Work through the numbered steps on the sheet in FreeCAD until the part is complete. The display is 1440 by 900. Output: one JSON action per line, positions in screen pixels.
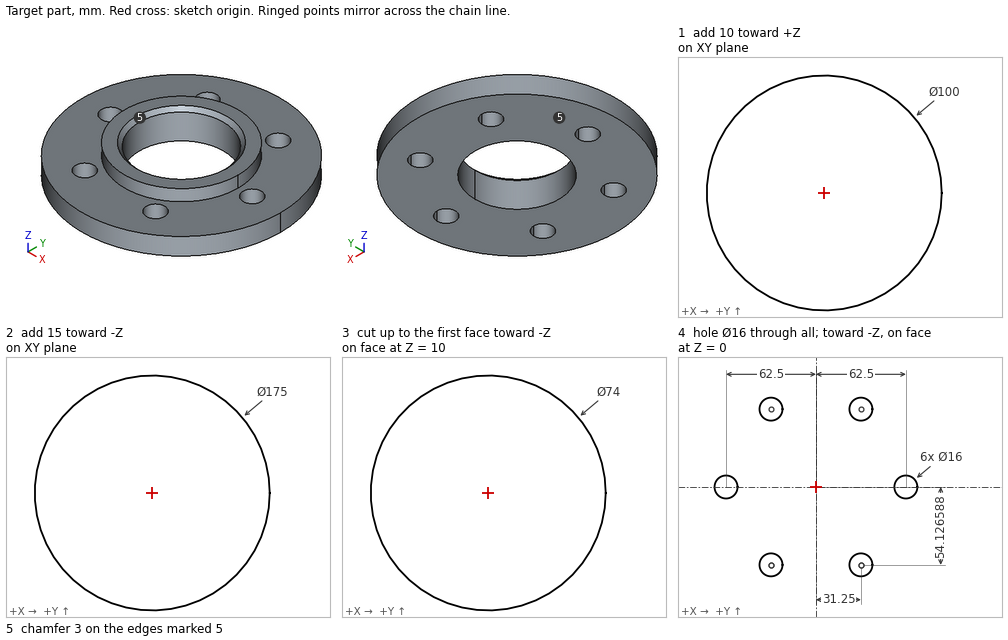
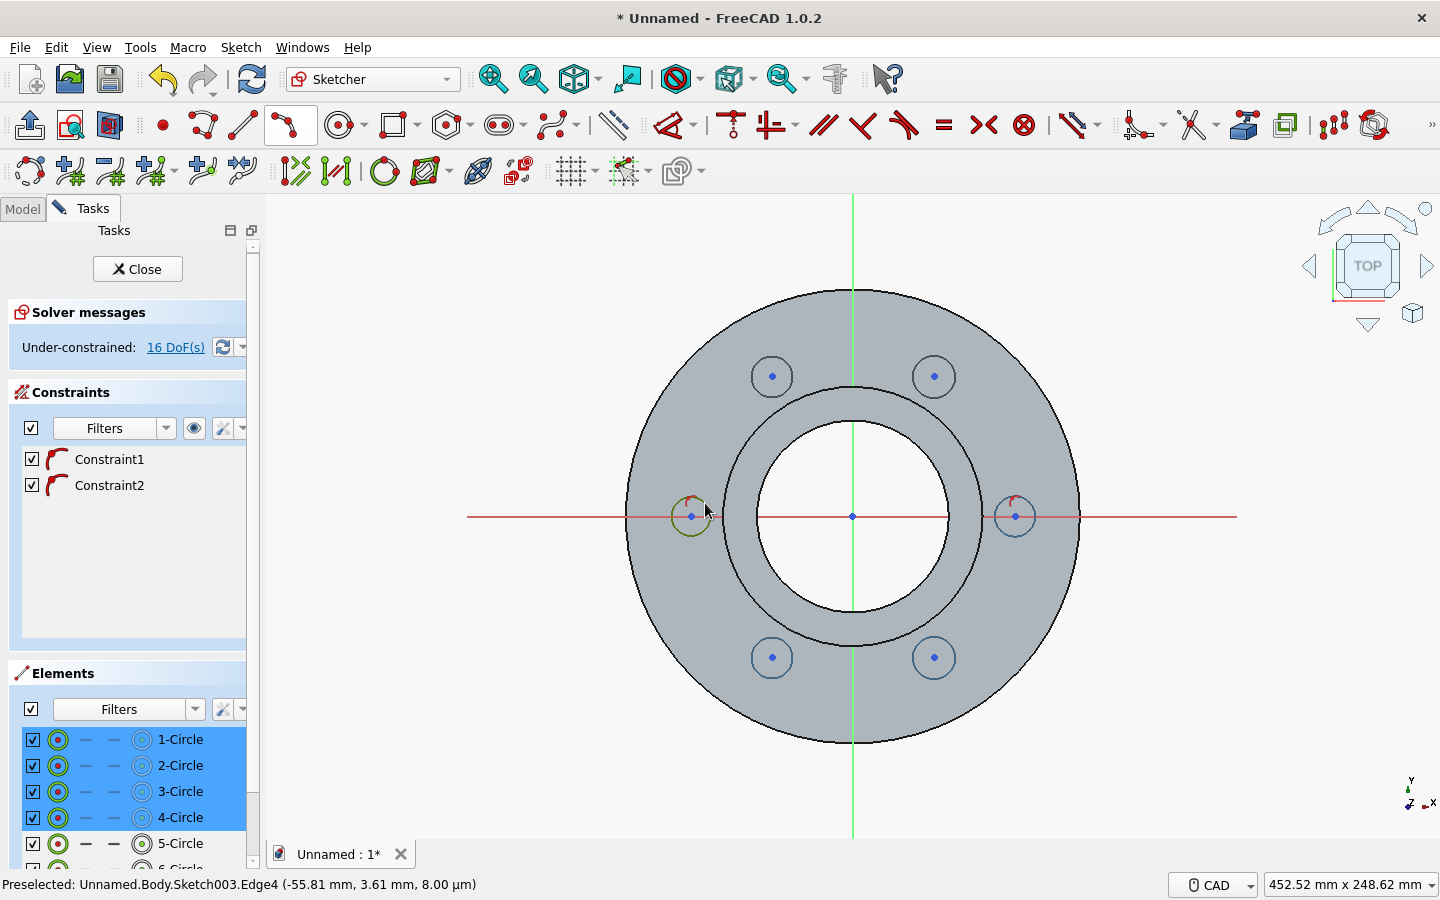
{"action": "left_click", "coordinate": [786, 362]}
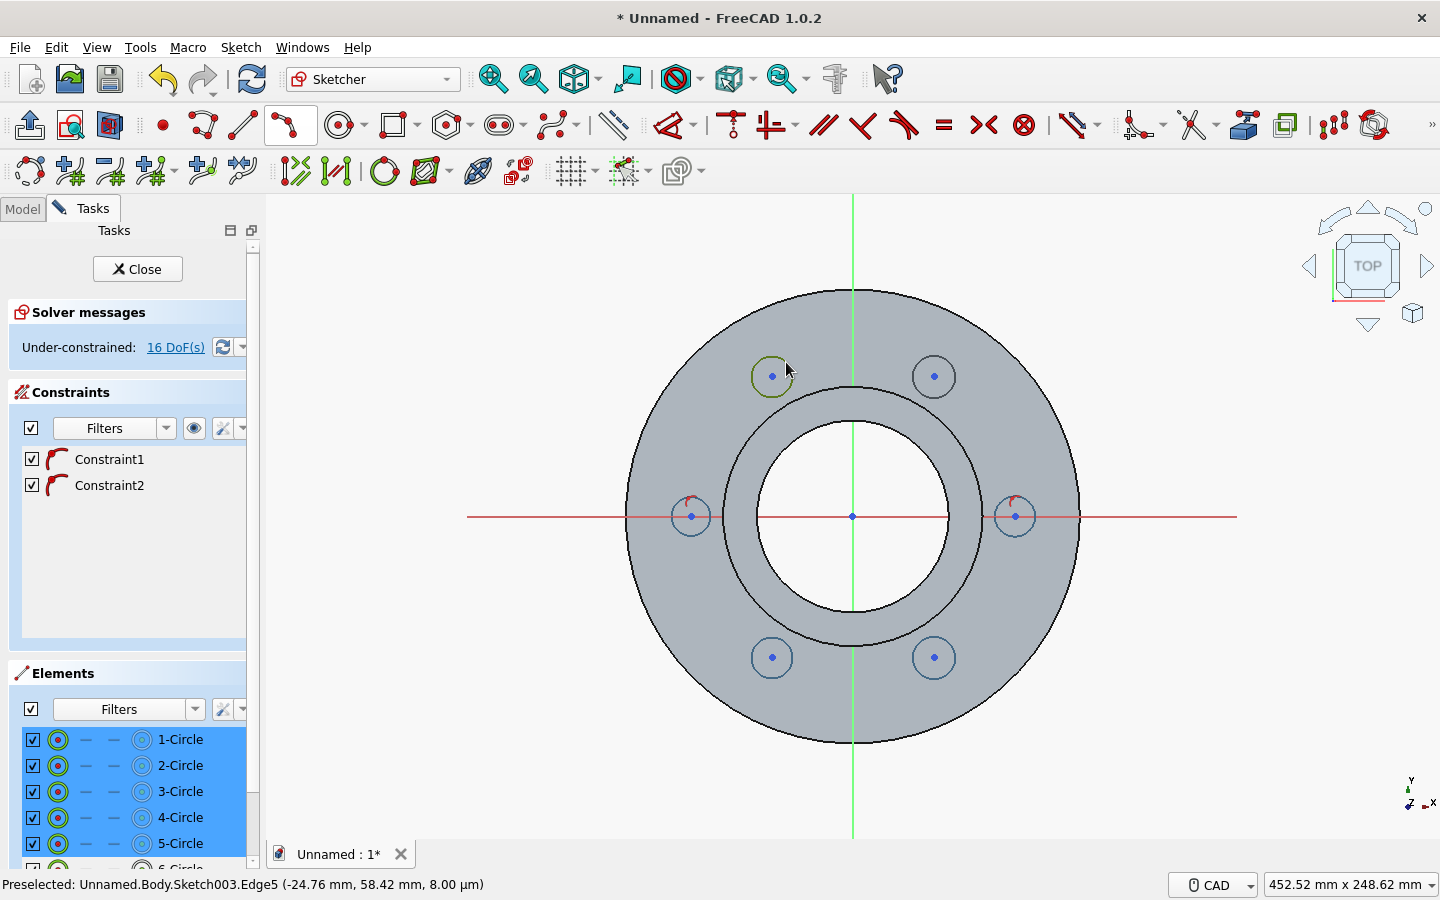
{"action": "left_click", "coordinate": [949, 362]}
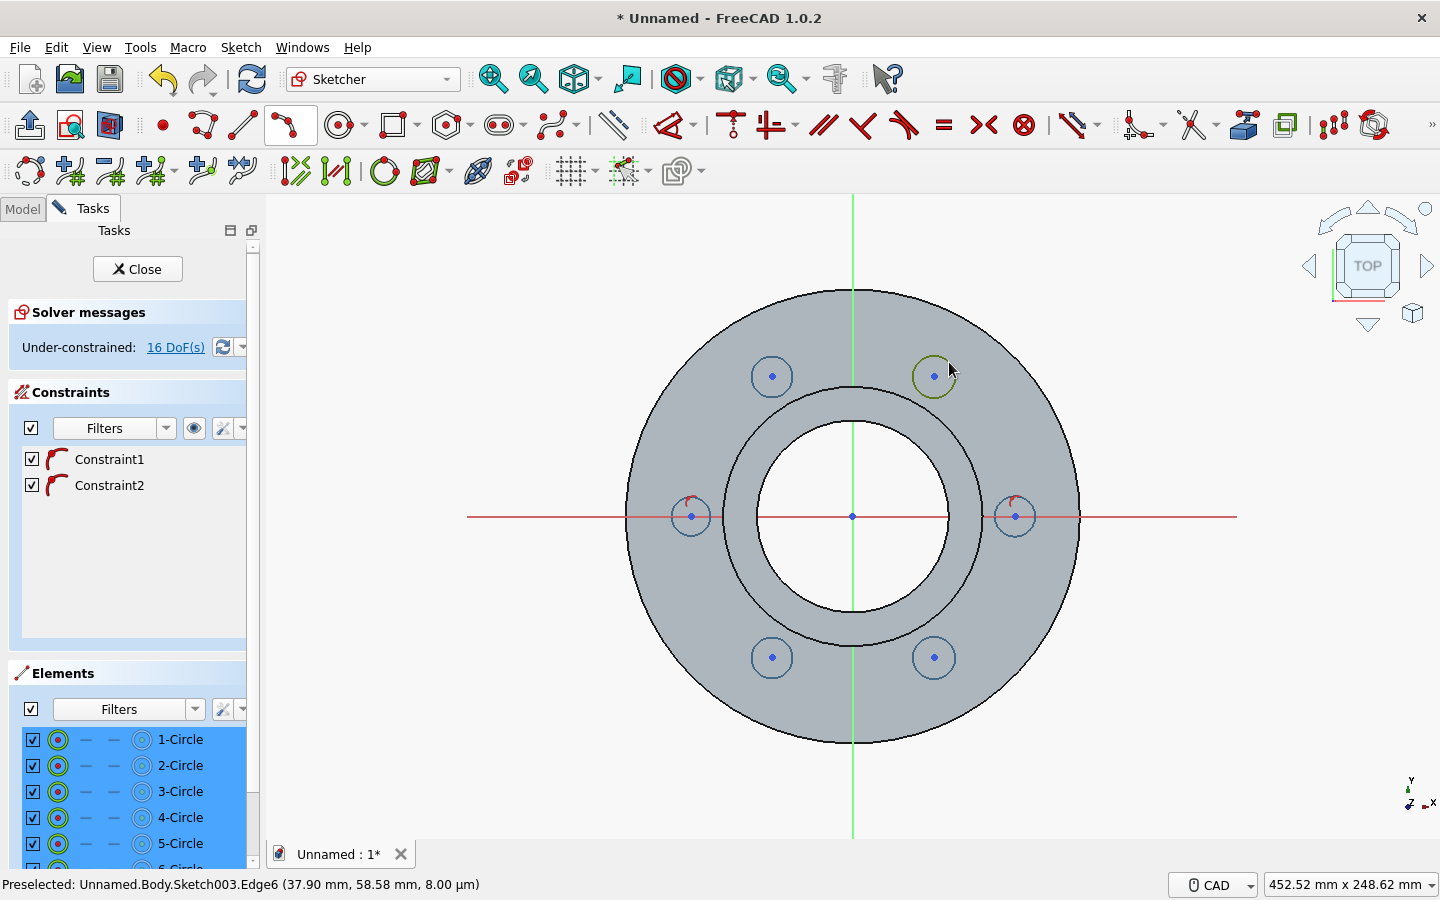
{"action": "key", "text": "e"}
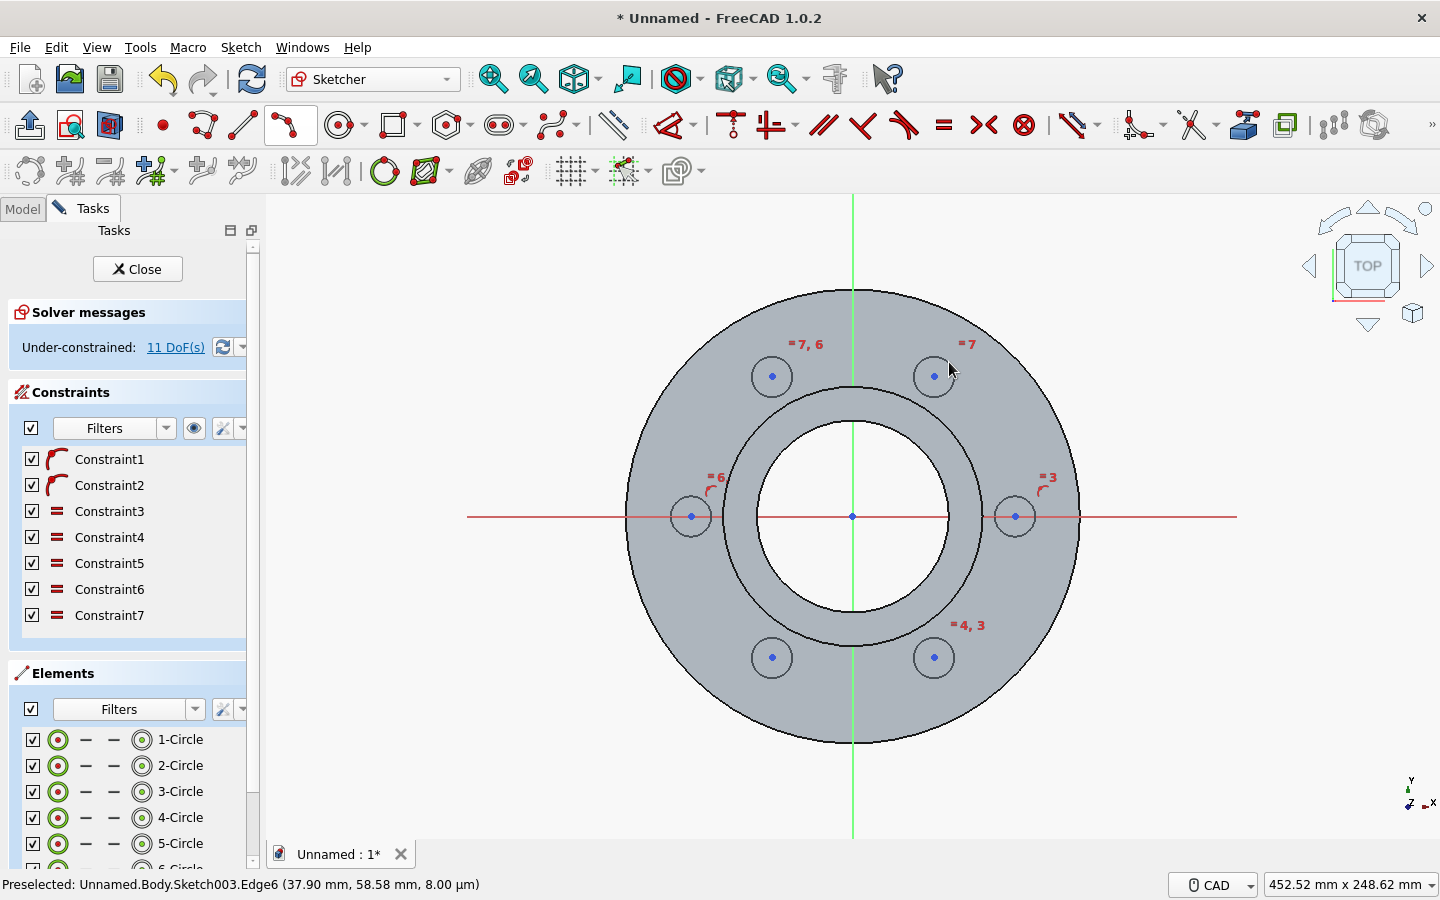
{"action": "left_click", "coordinate": [934, 658]}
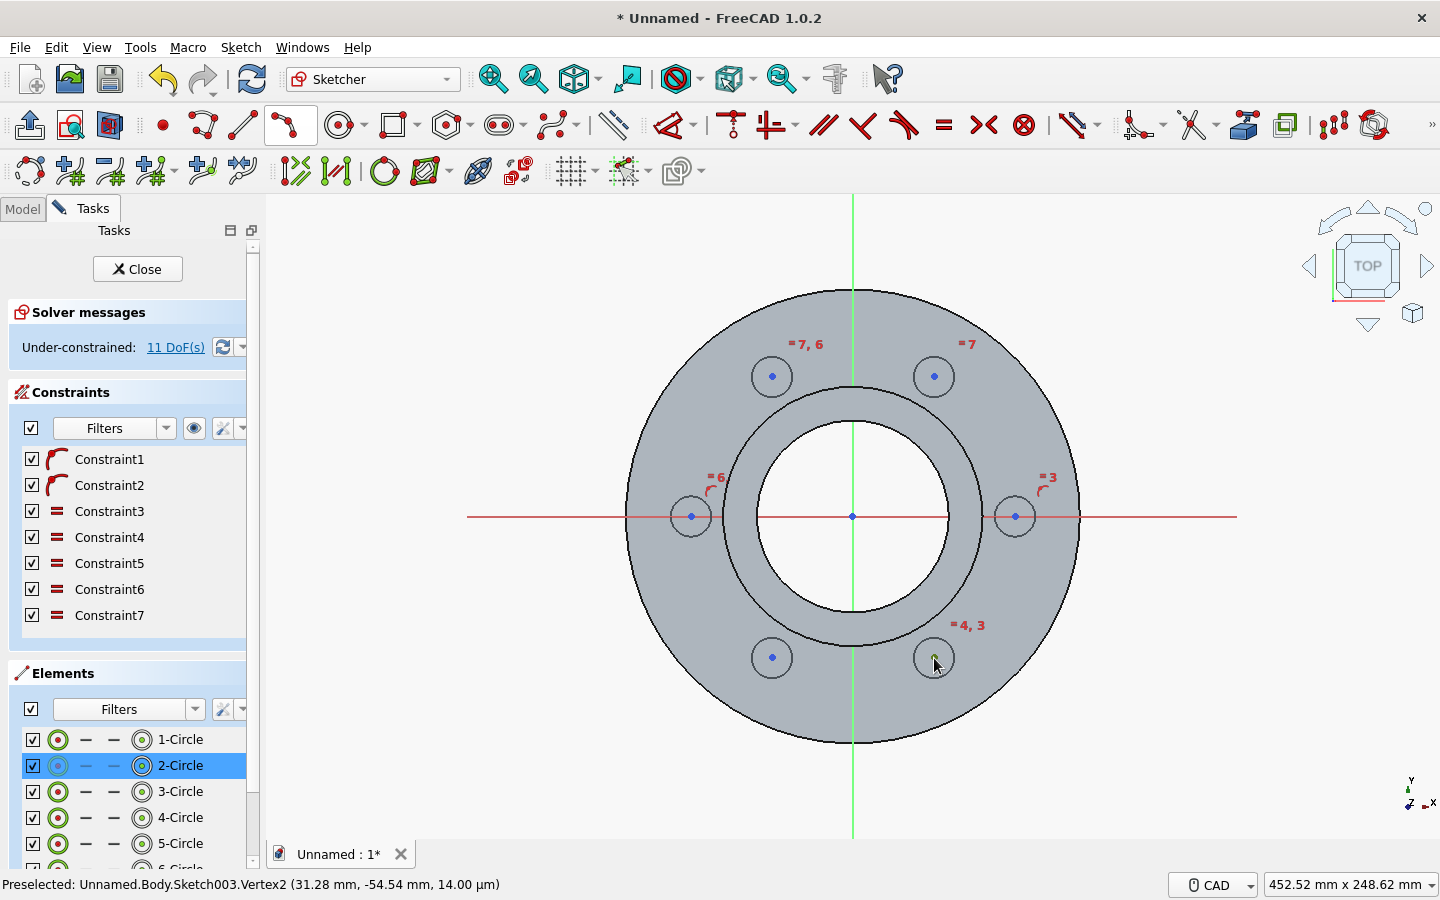
{"action": "left_click", "coordinate": [772, 658]}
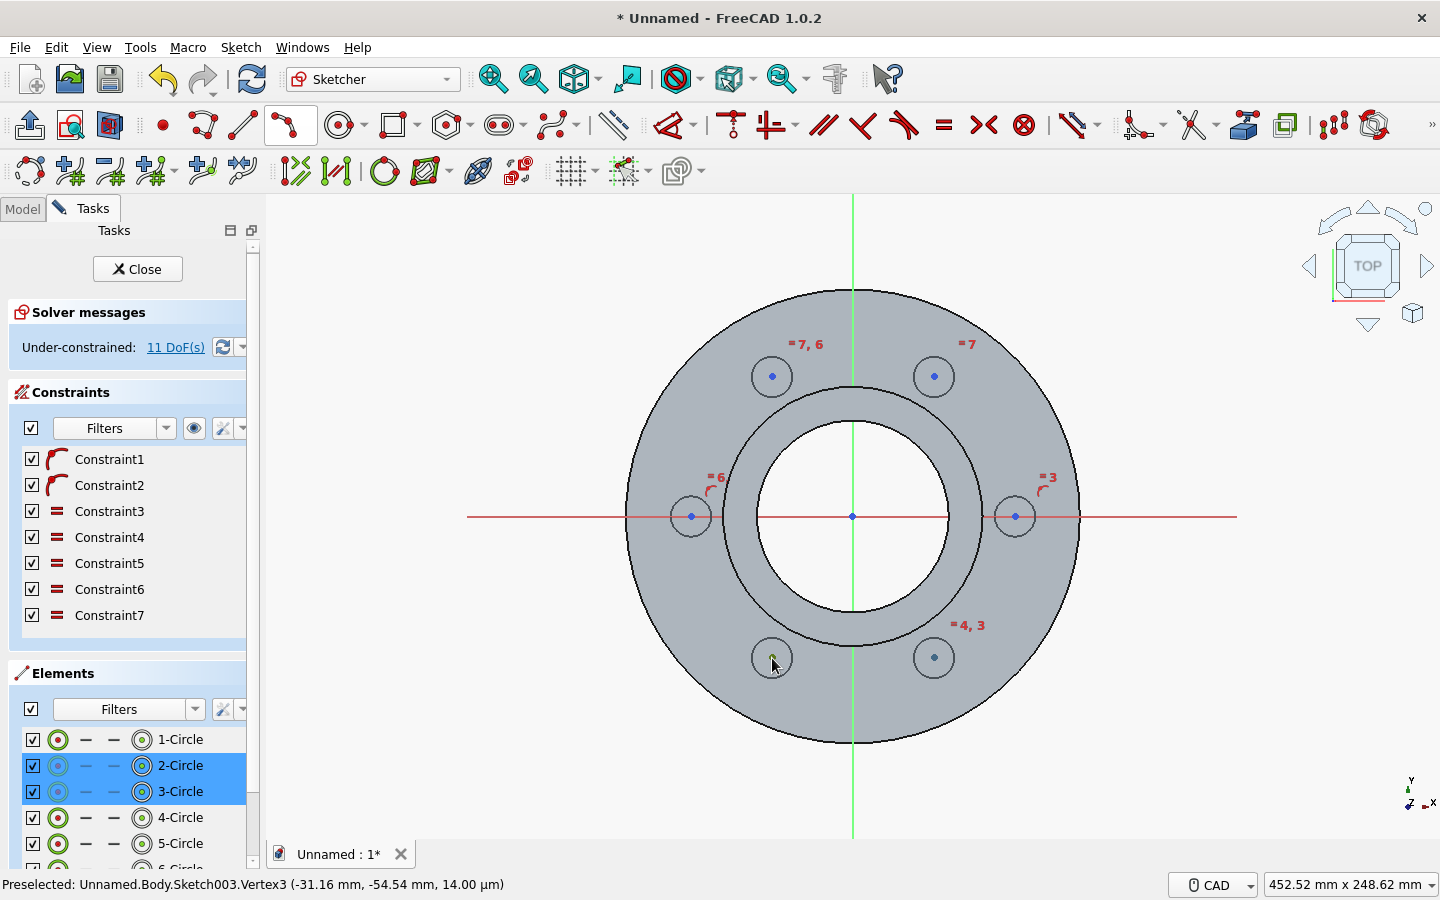
{"action": "left_click", "coordinate": [853, 769]}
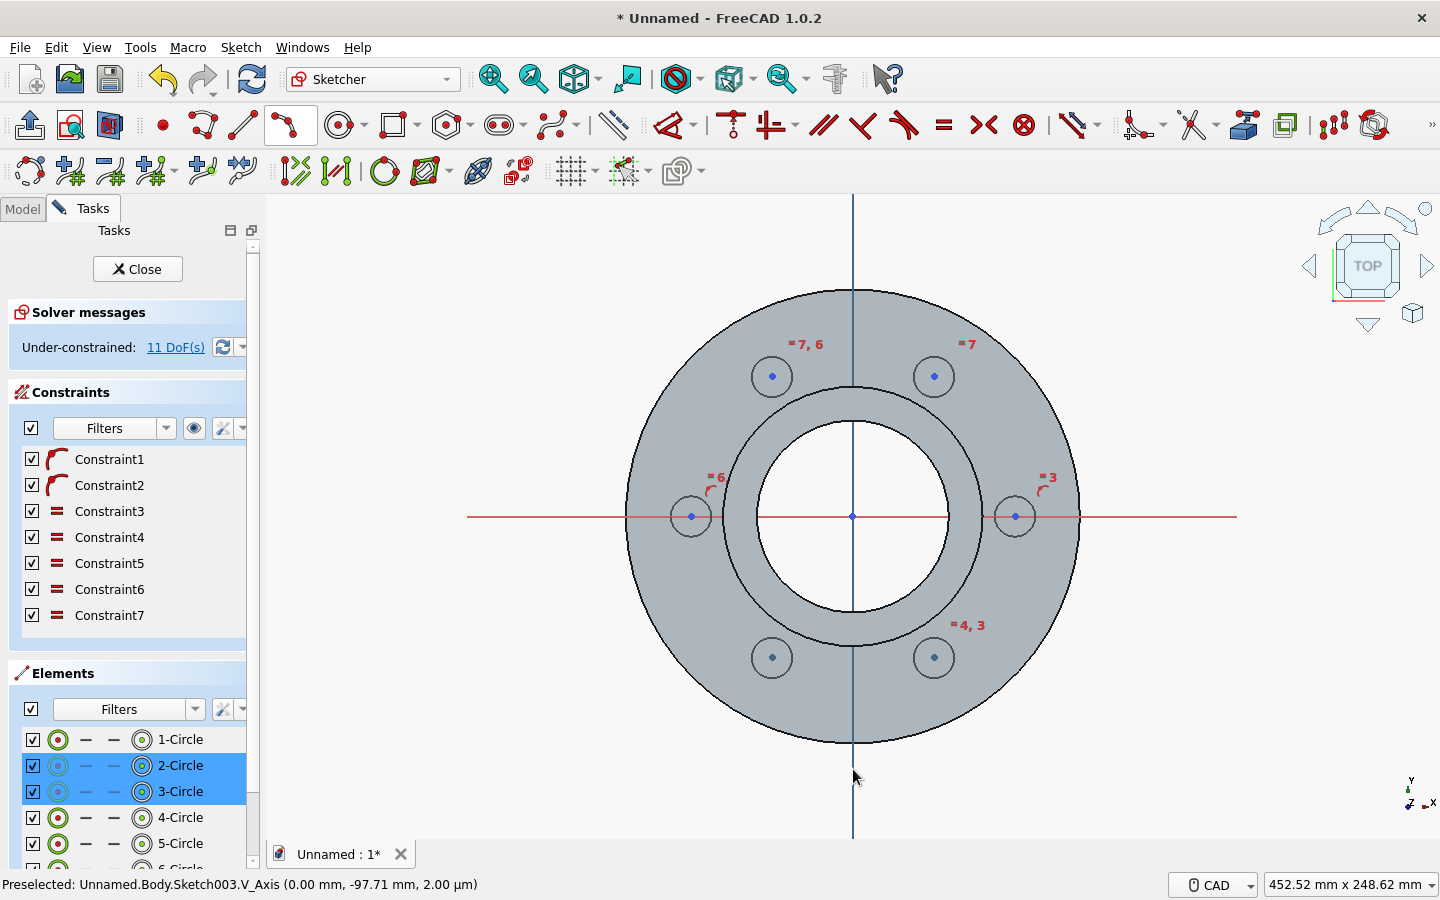
{"action": "left_click", "coordinate": [984, 126]}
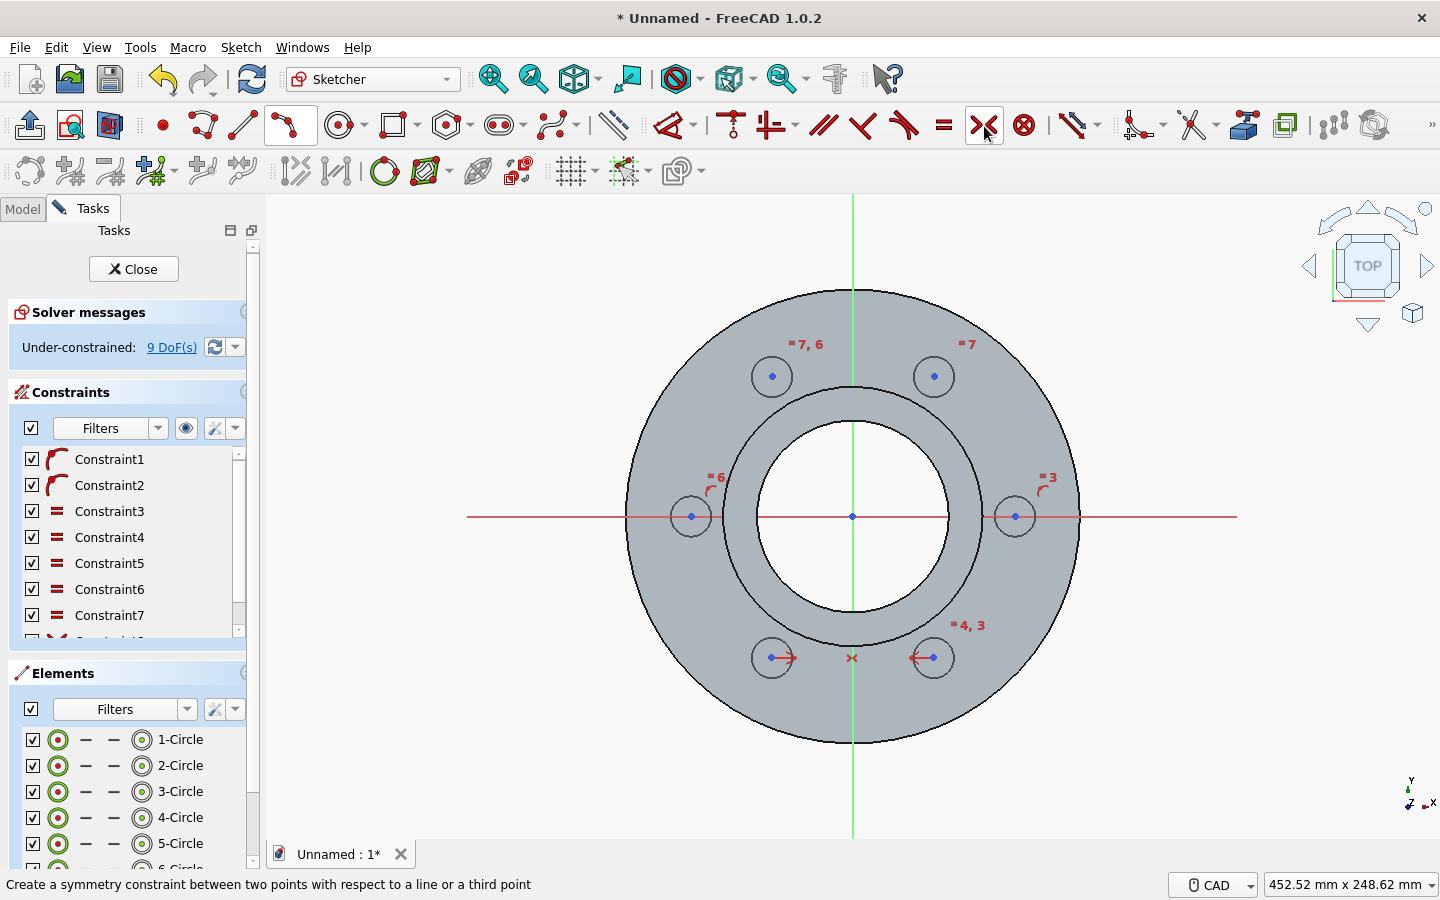
{"action": "left_click", "coordinate": [772, 658]}